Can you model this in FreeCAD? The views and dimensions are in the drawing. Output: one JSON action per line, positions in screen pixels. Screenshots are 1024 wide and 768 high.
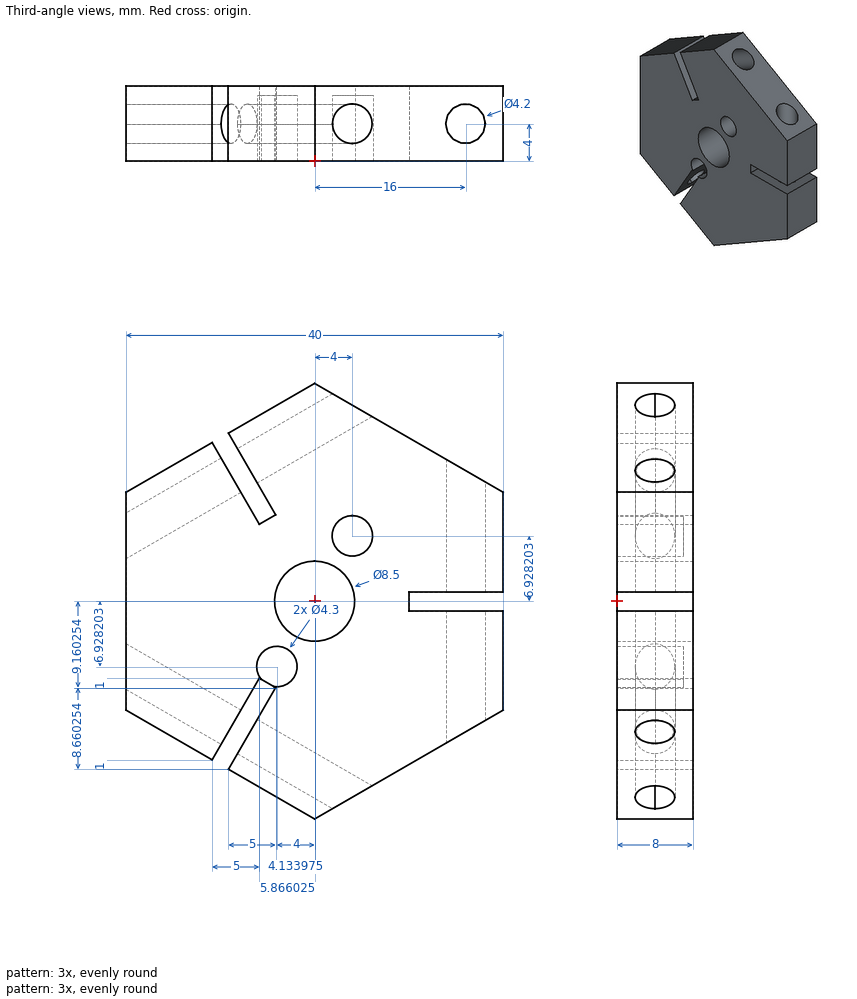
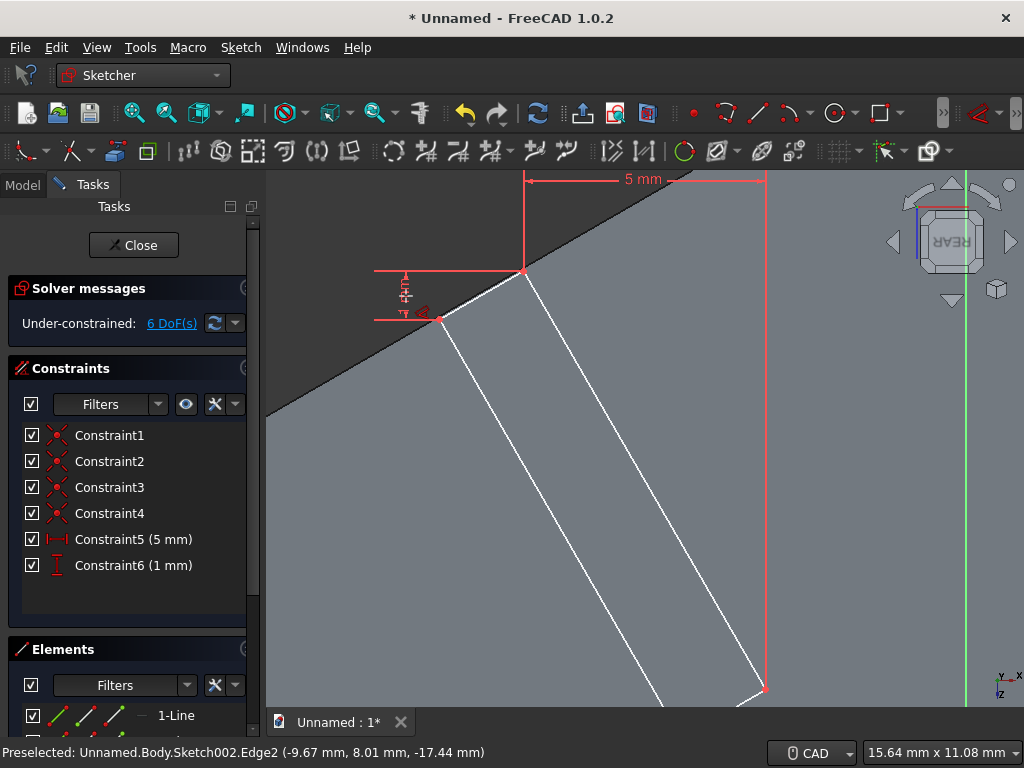
{"action": "left_click", "coordinate": [512, 445]}
{"action": "left_click", "coordinate": [561, 286]}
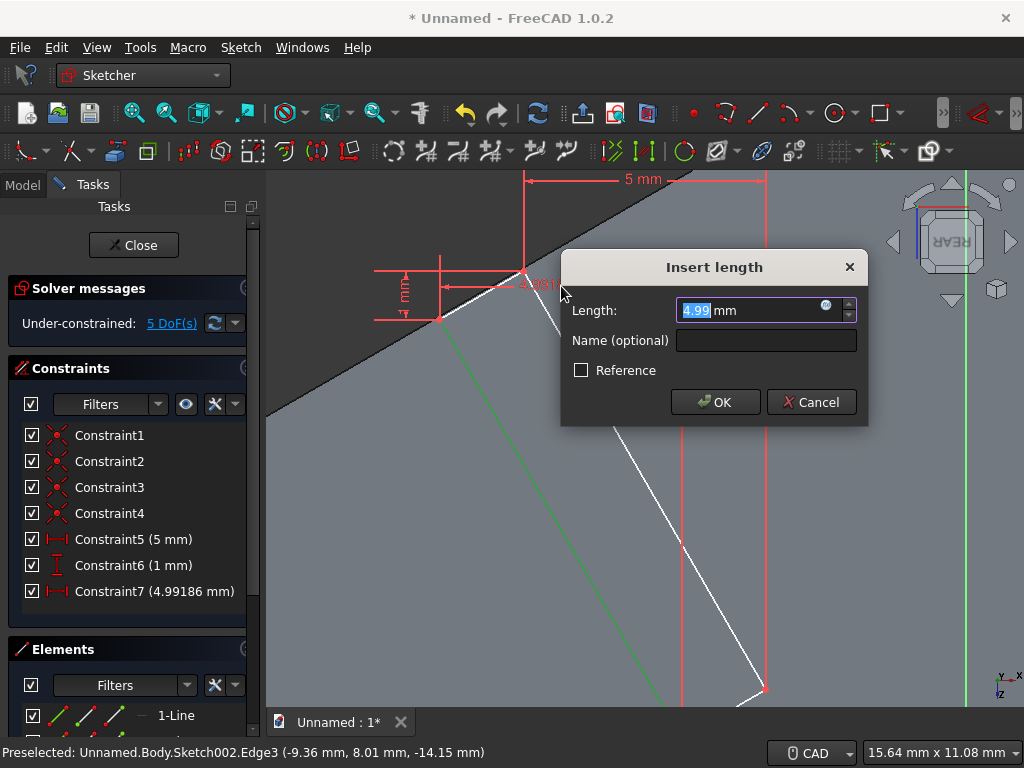
{"action": "type", "text": "5"}
{"action": "key", "text": "Return"}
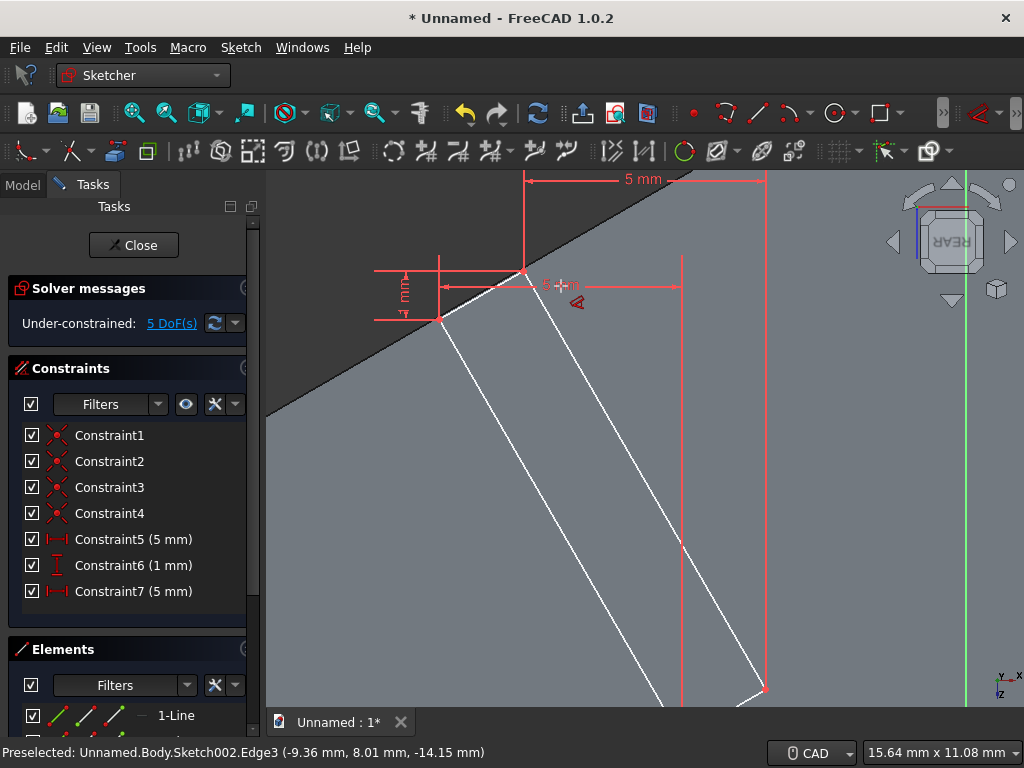
{"action": "scroll", "coordinate": [503, 286], "scroll_direction": "down", "scroll_amount": 5}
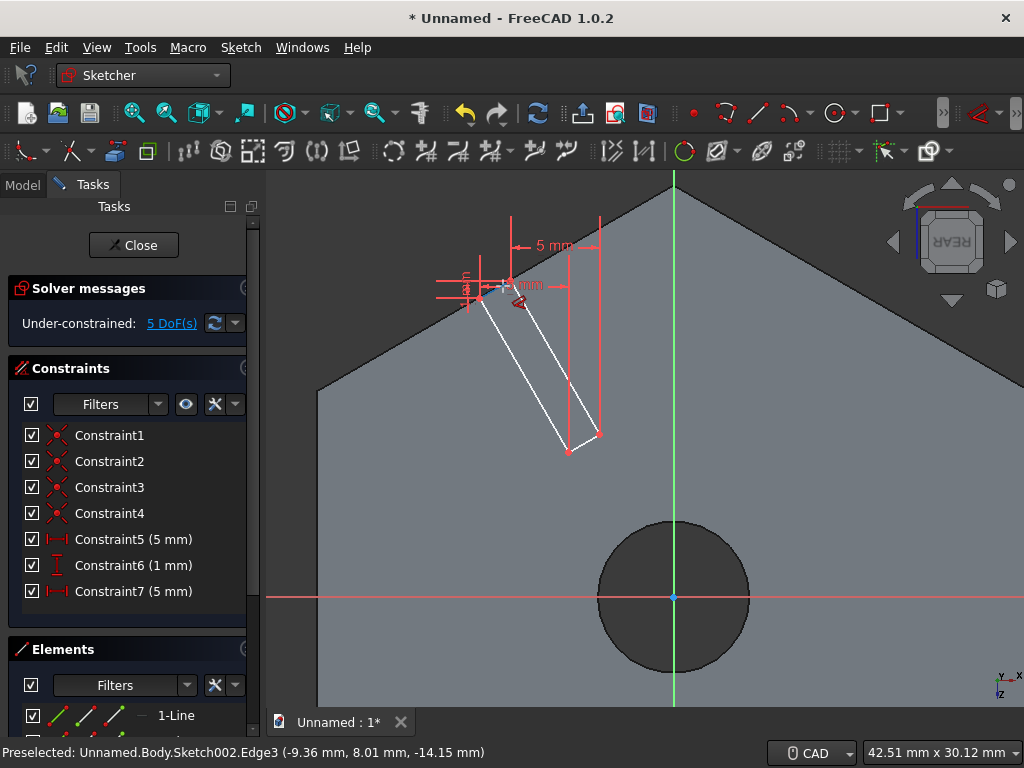
{"action": "scroll", "coordinate": [578, 447], "scroll_direction": "up", "scroll_amount": 5}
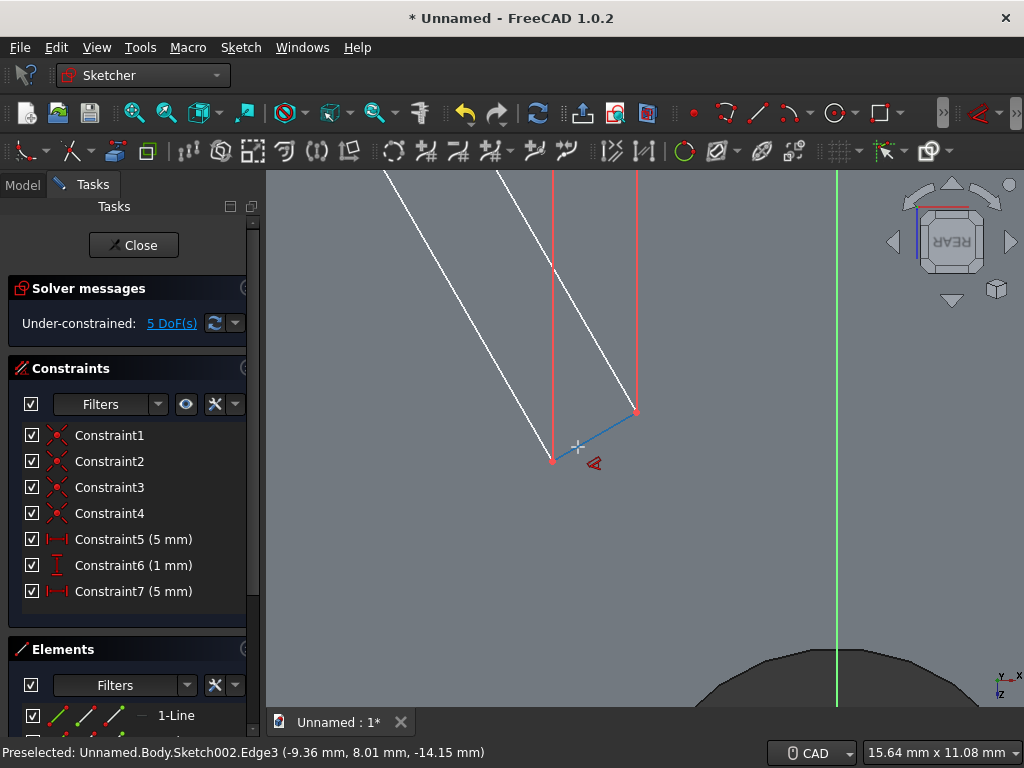
{"action": "left_click", "coordinate": [578, 447]}
{"action": "left_click", "coordinate": [671, 437]}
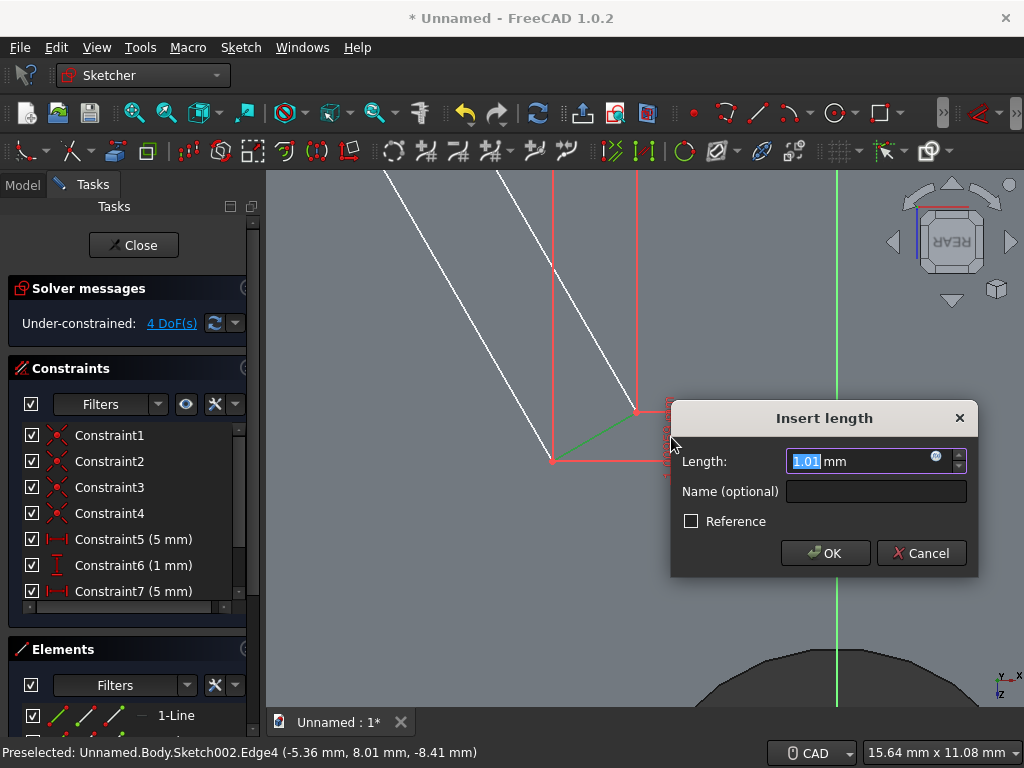
{"action": "type", "text": "1"}
{"action": "key", "text": "Return"}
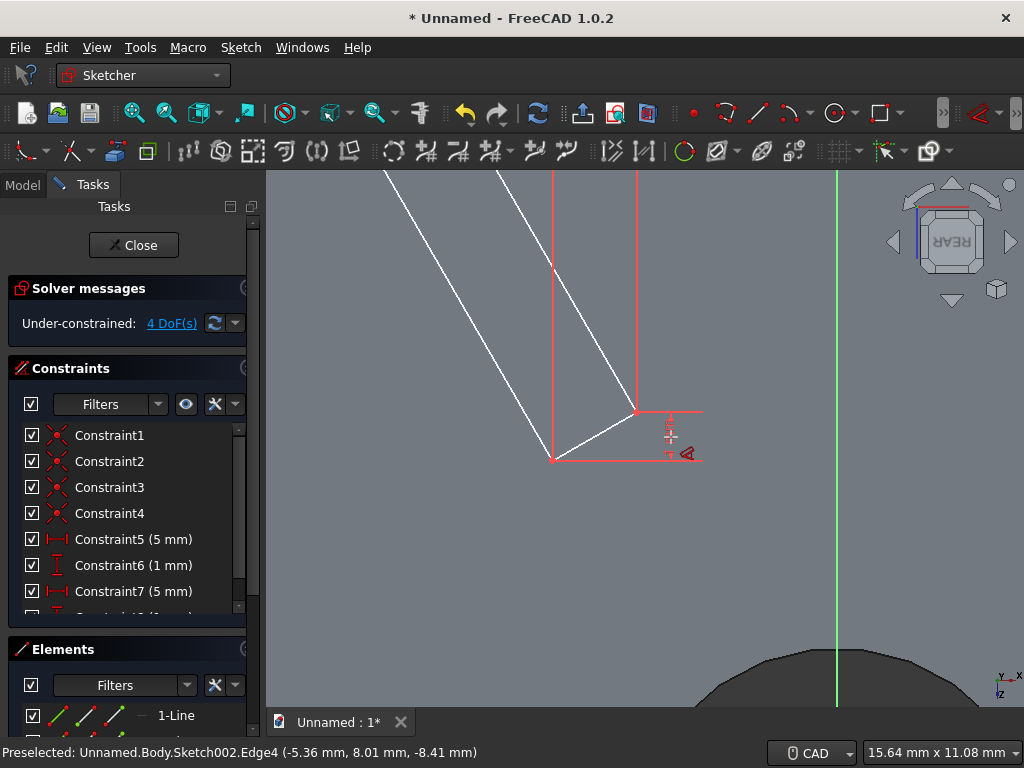
{"action": "left_click", "coordinate": [637, 412]}
{"action": "left_click", "coordinate": [737, 378]}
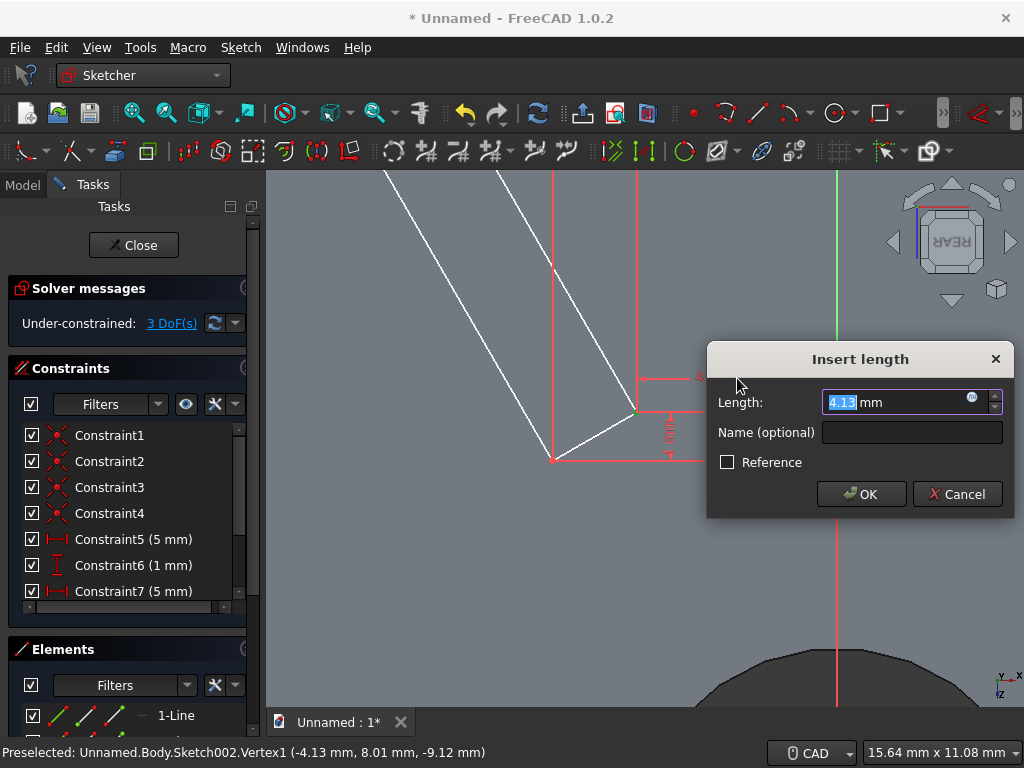
{"action": "type", "text": "4.133975"}
{"action": "key", "text": "Return"}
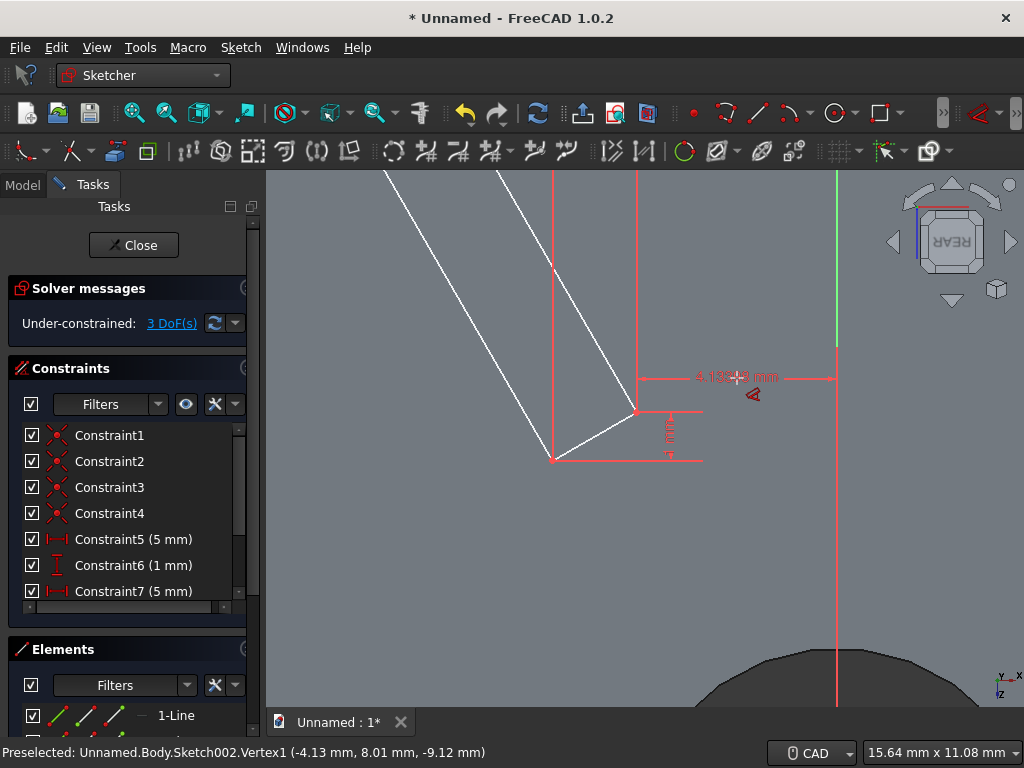
{"action": "left_click", "coordinate": [637, 412]}
{"action": "left_click", "coordinate": [603, 546]}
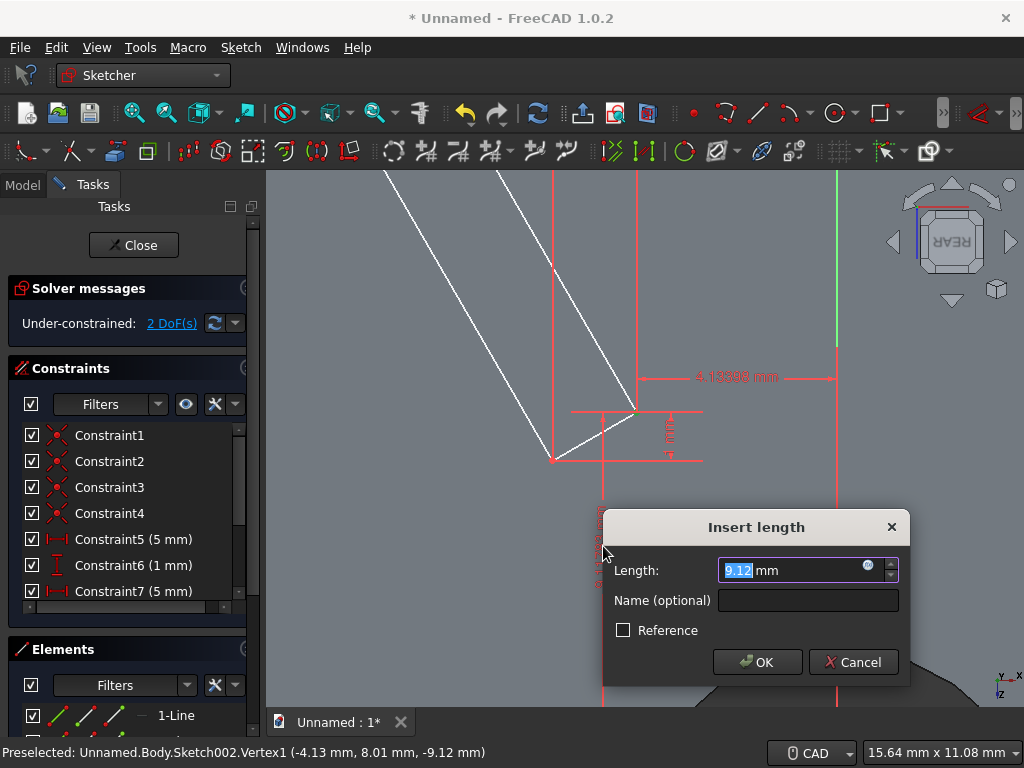
{"action": "type", "text": "9.160254"}
{"action": "key", "text": "Return"}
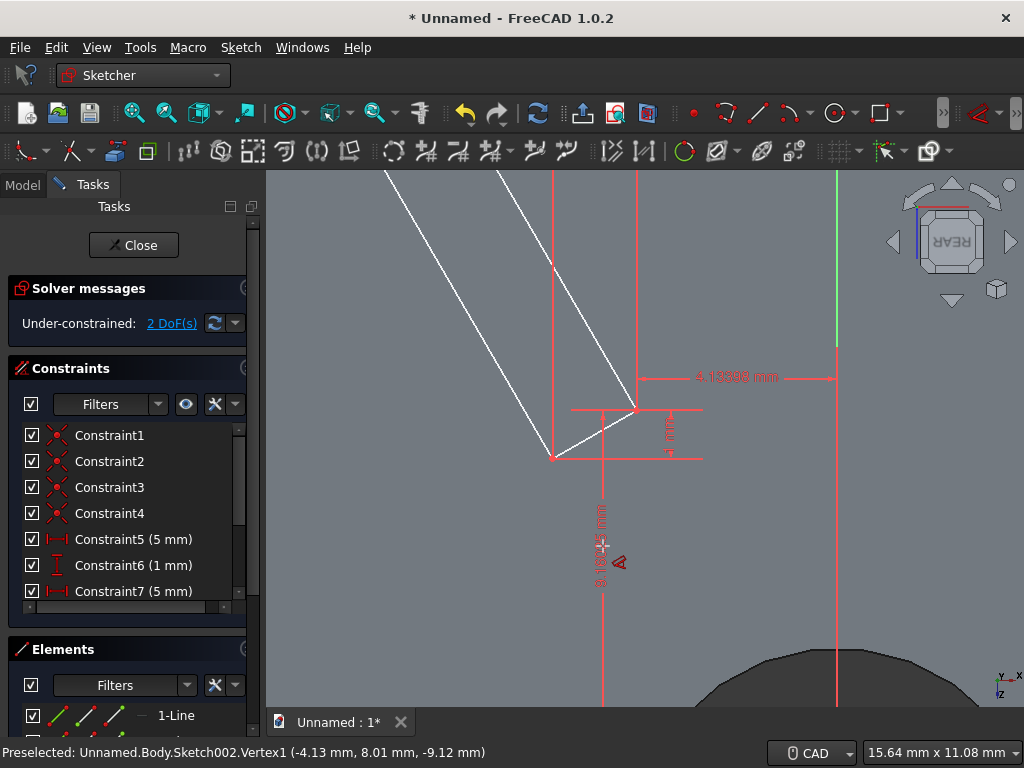
{"action": "left_click", "coordinate": [553, 459]}
{"action": "left_click", "coordinate": [760, 425]}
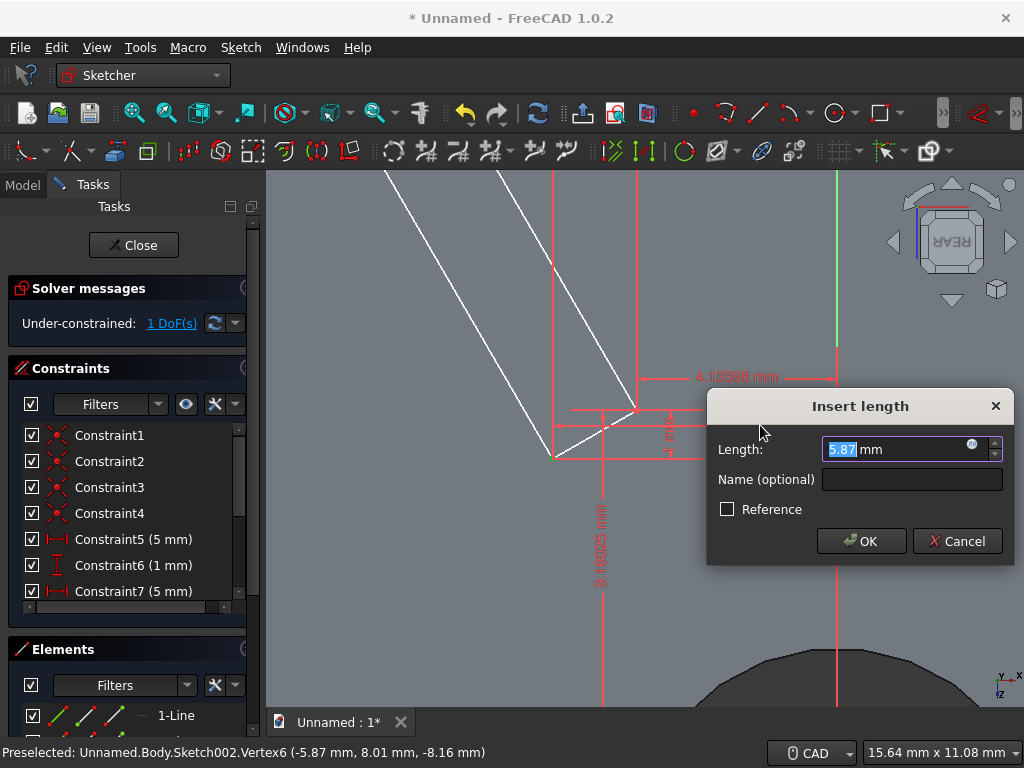
{"action": "type", "text": "5.866025"}
{"action": "key", "text": "Return"}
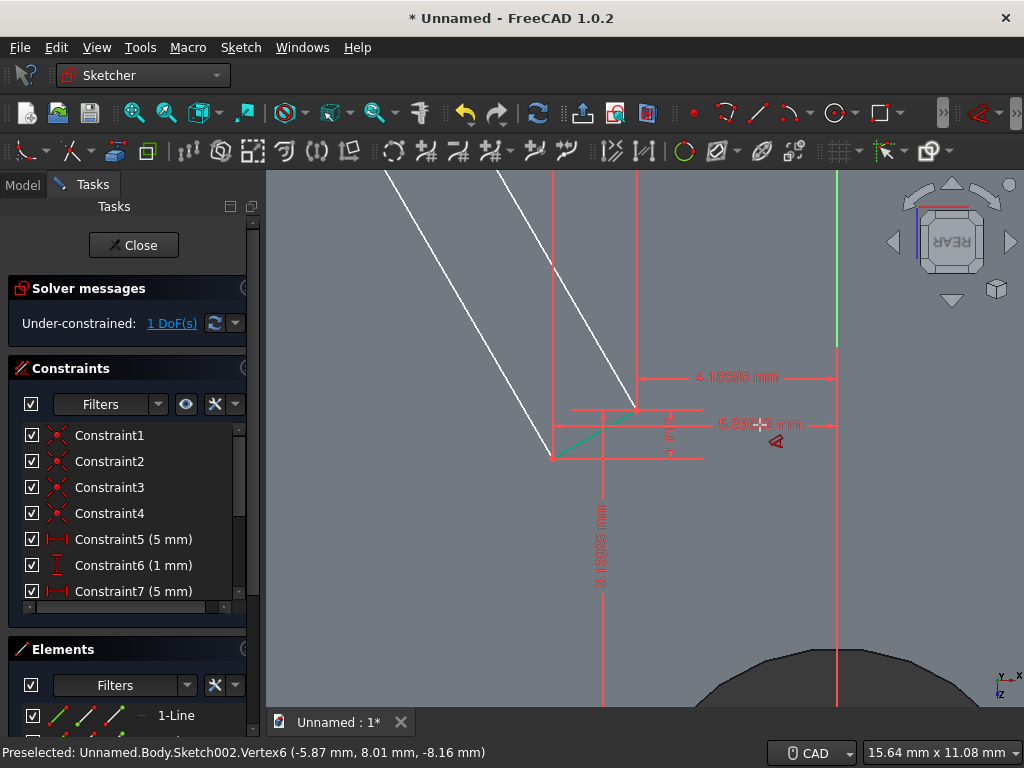
{"action": "left_click", "coordinate": [564, 285]}
{"action": "left_click", "coordinate": [361, 304]}